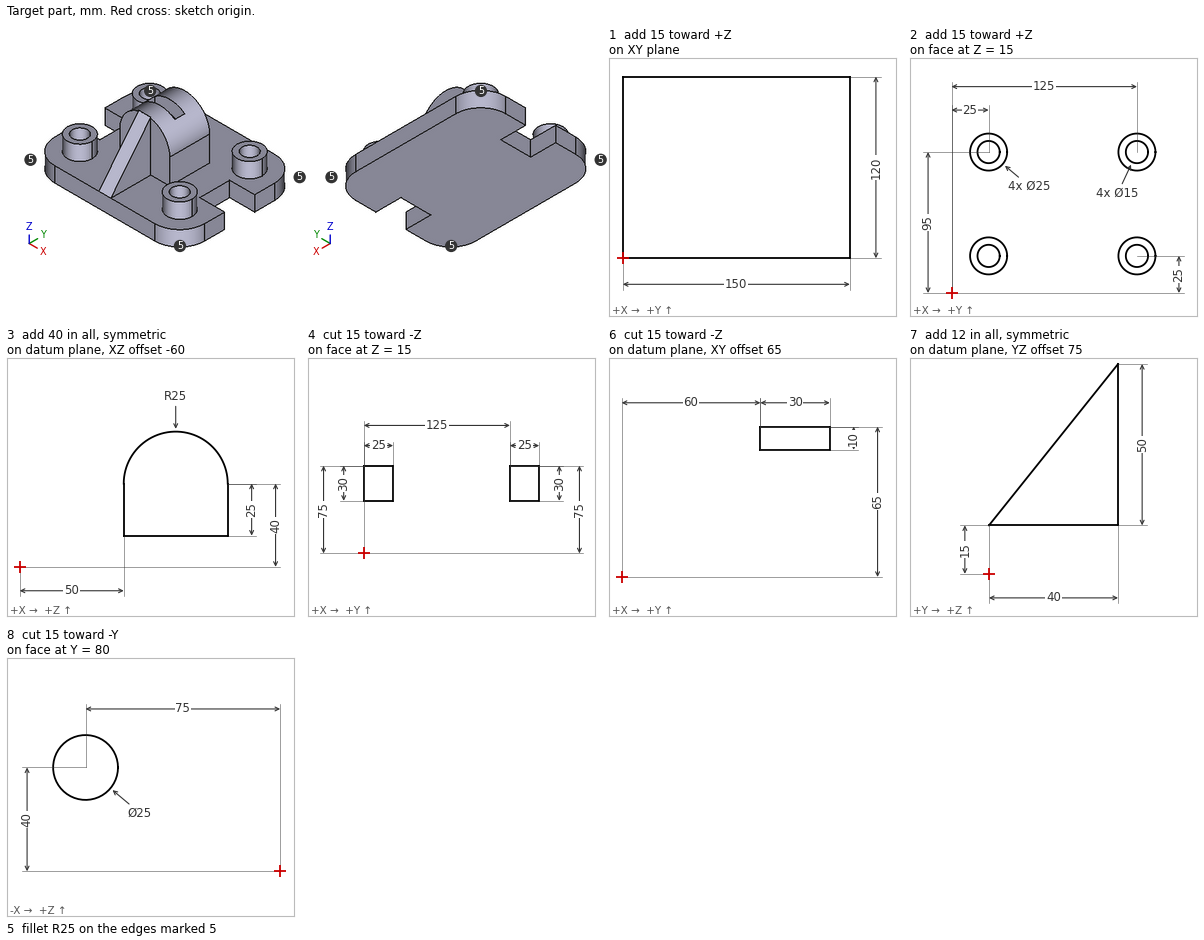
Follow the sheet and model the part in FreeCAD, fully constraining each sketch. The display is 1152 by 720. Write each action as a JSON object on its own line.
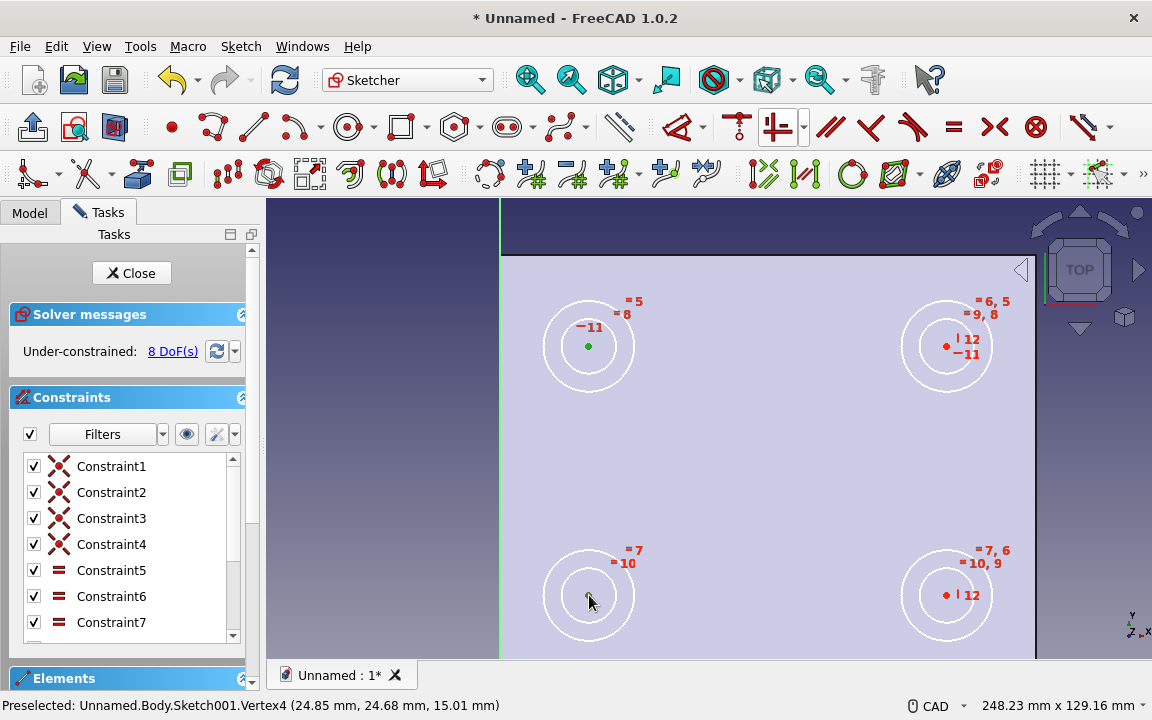
{"action": "key", "text": "v"}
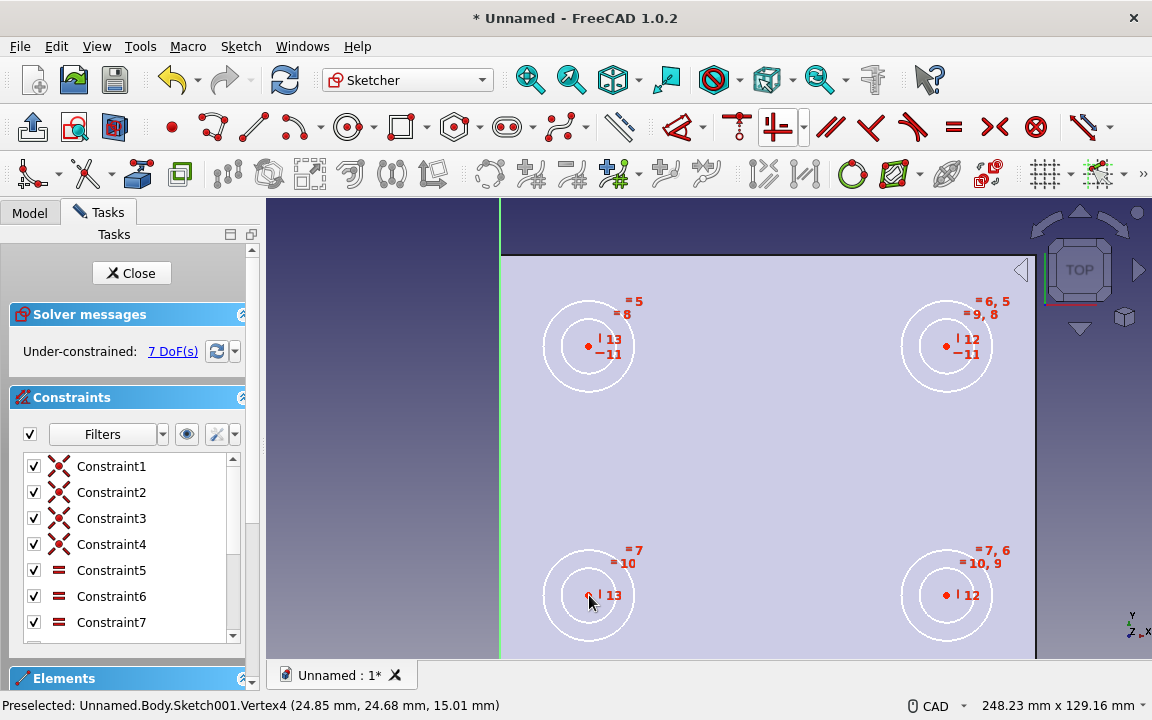
{"action": "left_click", "coordinate": [947, 595]}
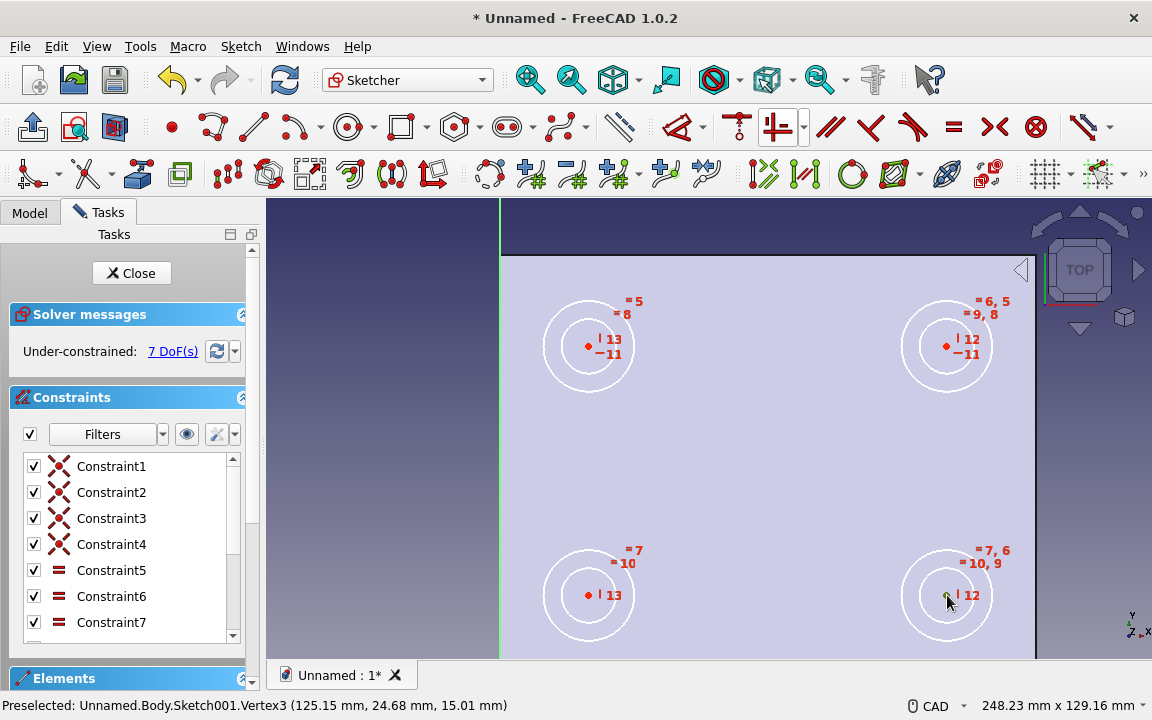
{"action": "left_click", "coordinate": [589, 595]}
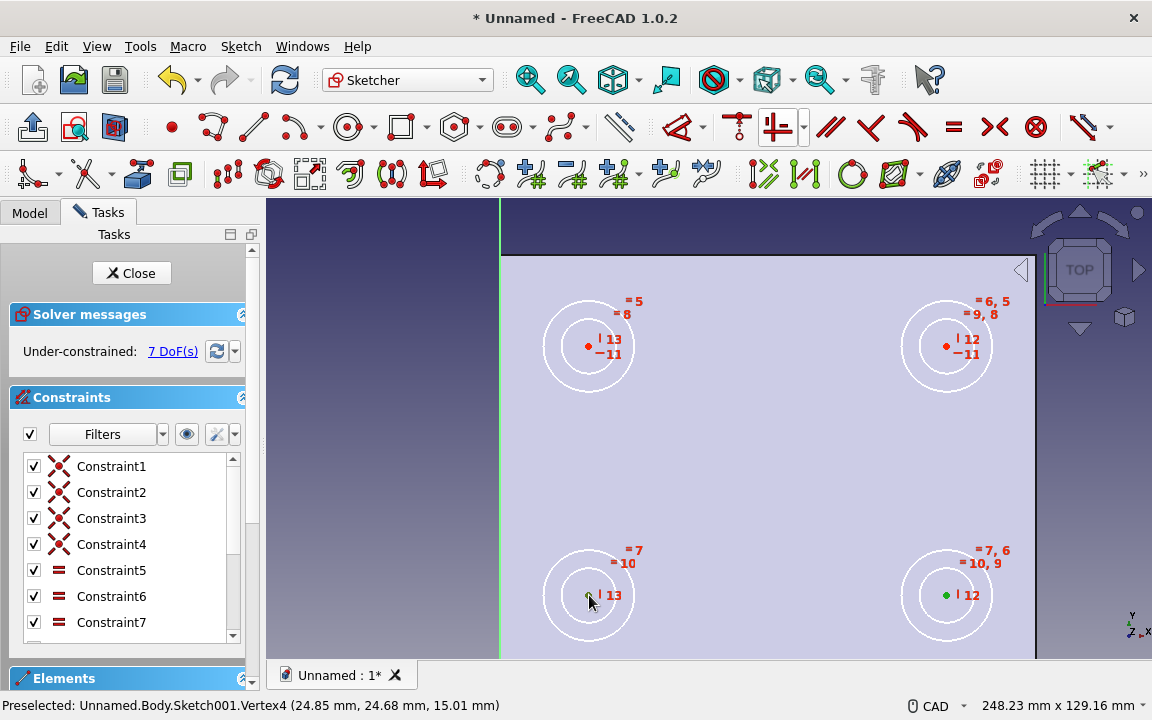
{"action": "key", "text": "h"}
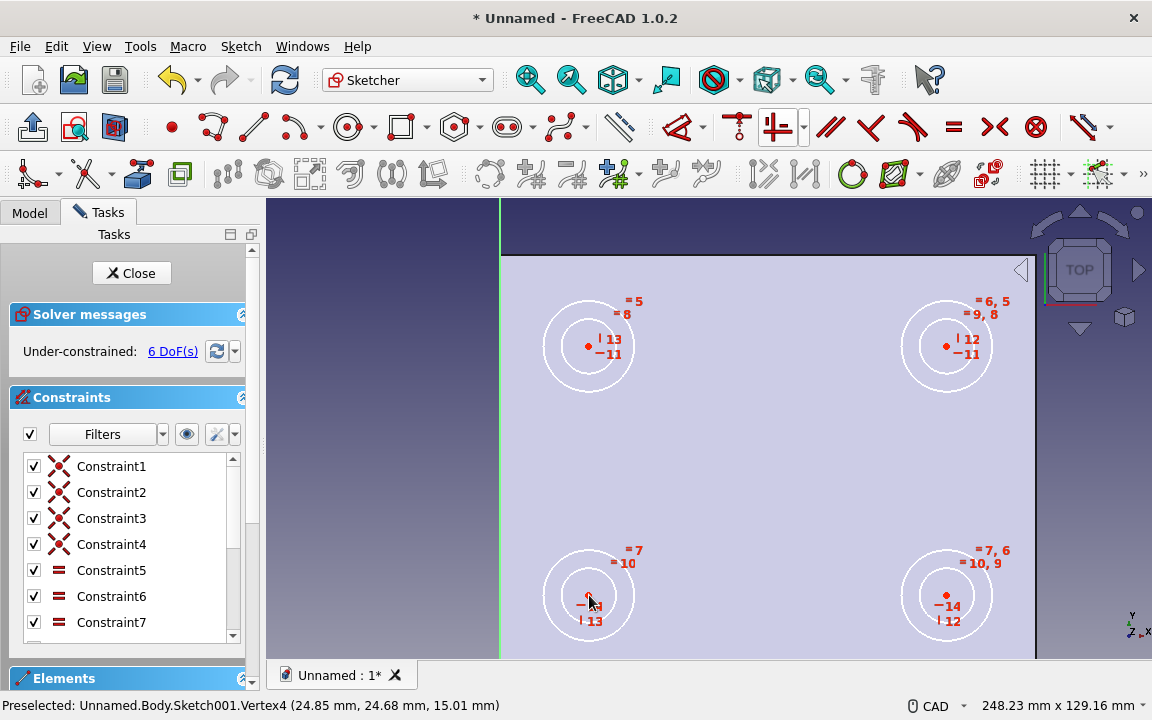
{"action": "left_click", "coordinate": [676, 128]}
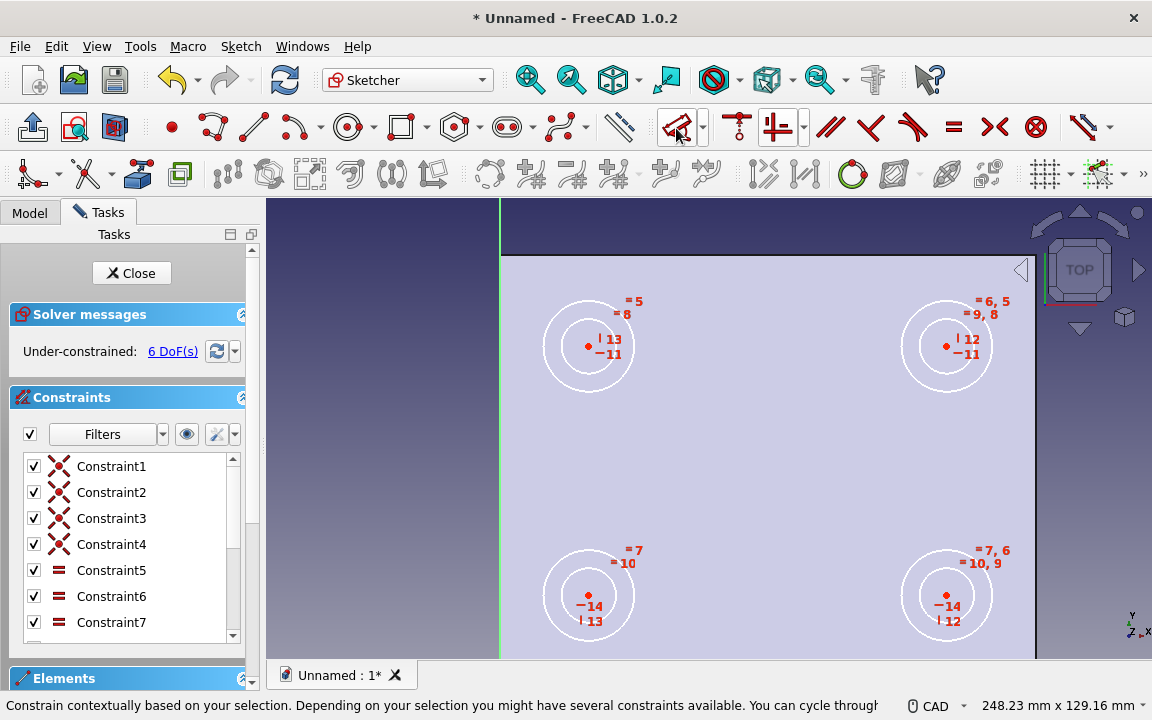
{"action": "left_click", "coordinate": [621, 314]}
{"action": "left_click", "coordinate": [644, 291]}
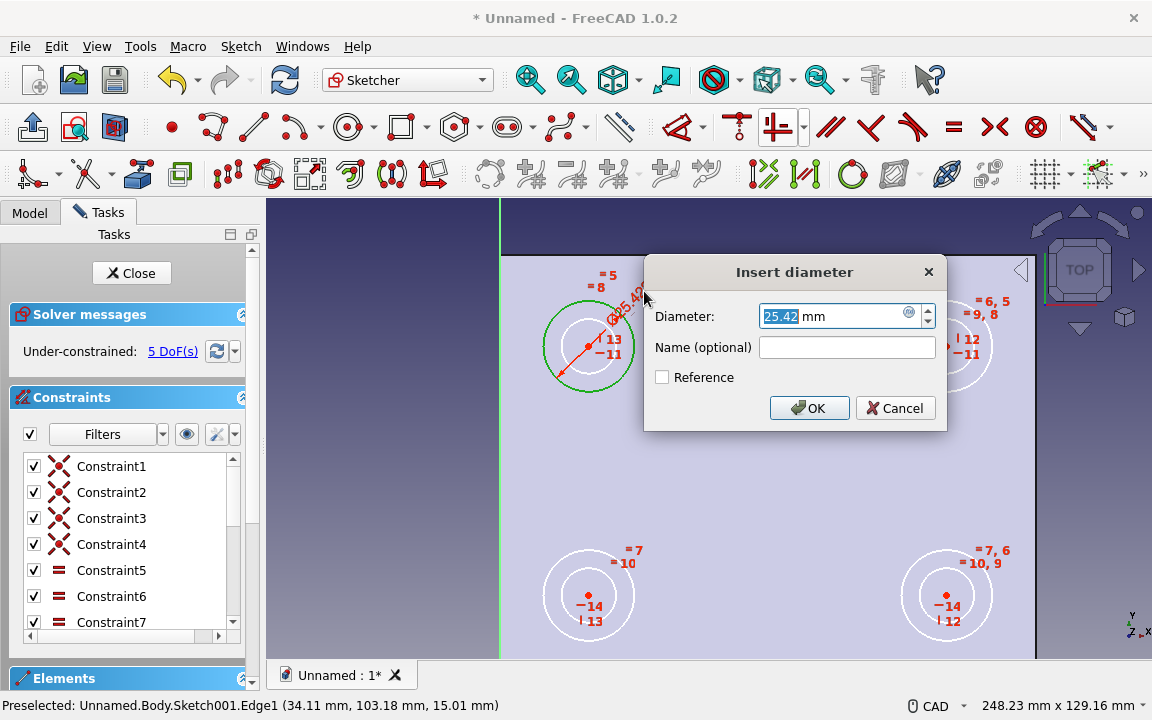
{"action": "type", "text": "25"}
{"action": "key", "text": "Return"}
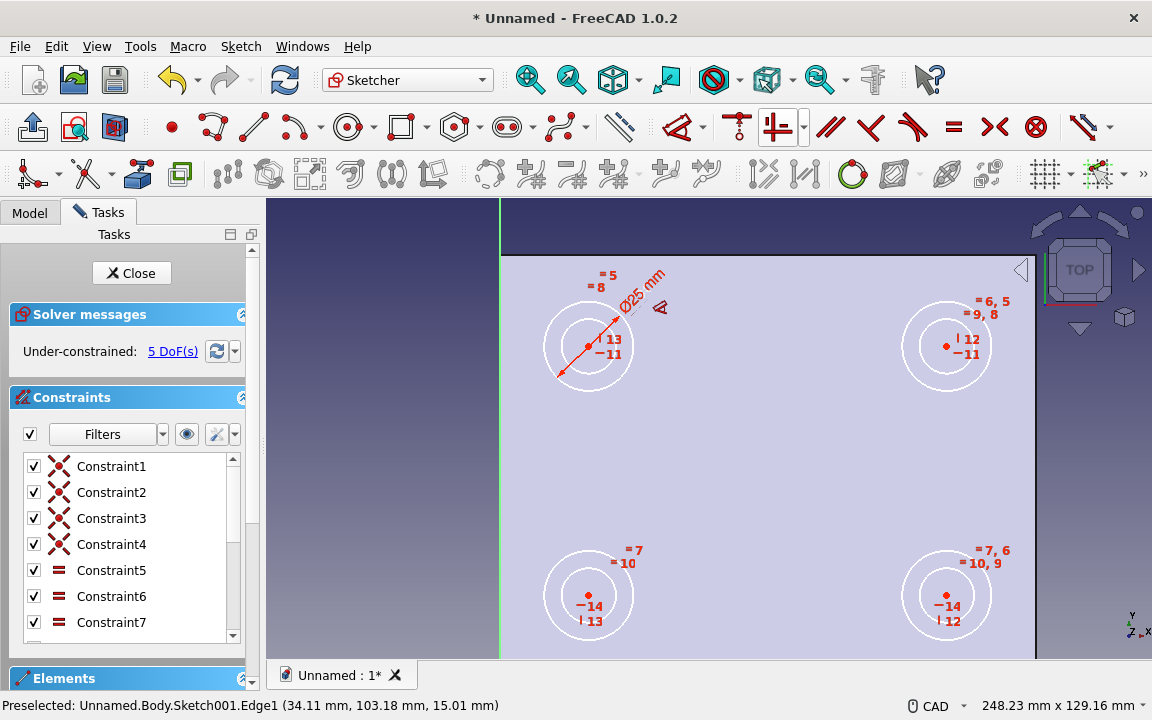
{"action": "left_click", "coordinate": [608, 327]}
{"action": "left_click", "coordinate": [646, 329]}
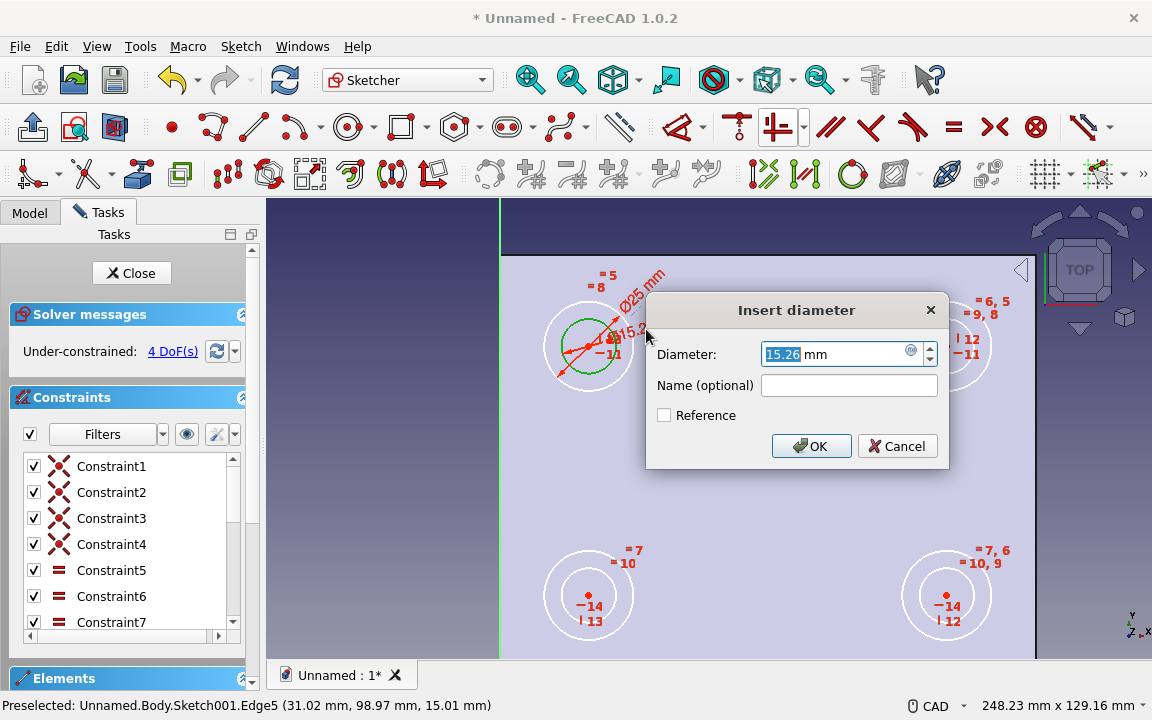
{"action": "type", "text": "15"}
{"action": "key", "text": "Return"}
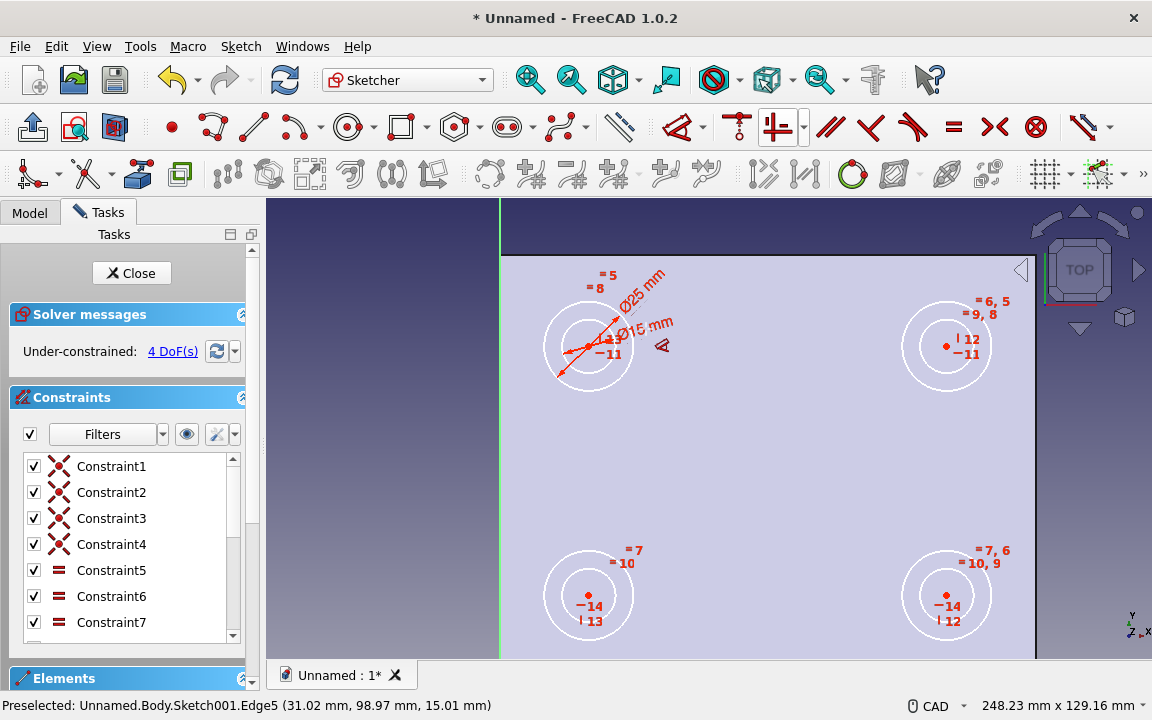
{"action": "left_click", "coordinate": [589, 346]}
{"action": "left_click", "coordinate": [524, 312]}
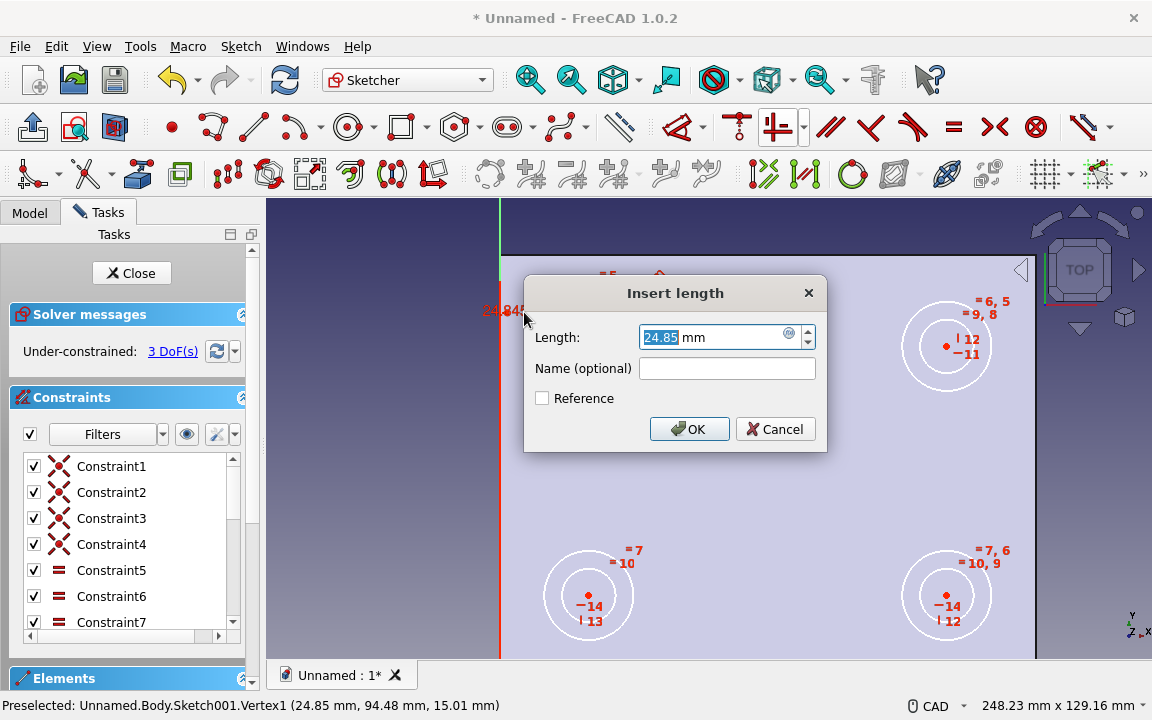
{"action": "type", "text": "25"}
{"action": "key", "text": "Return"}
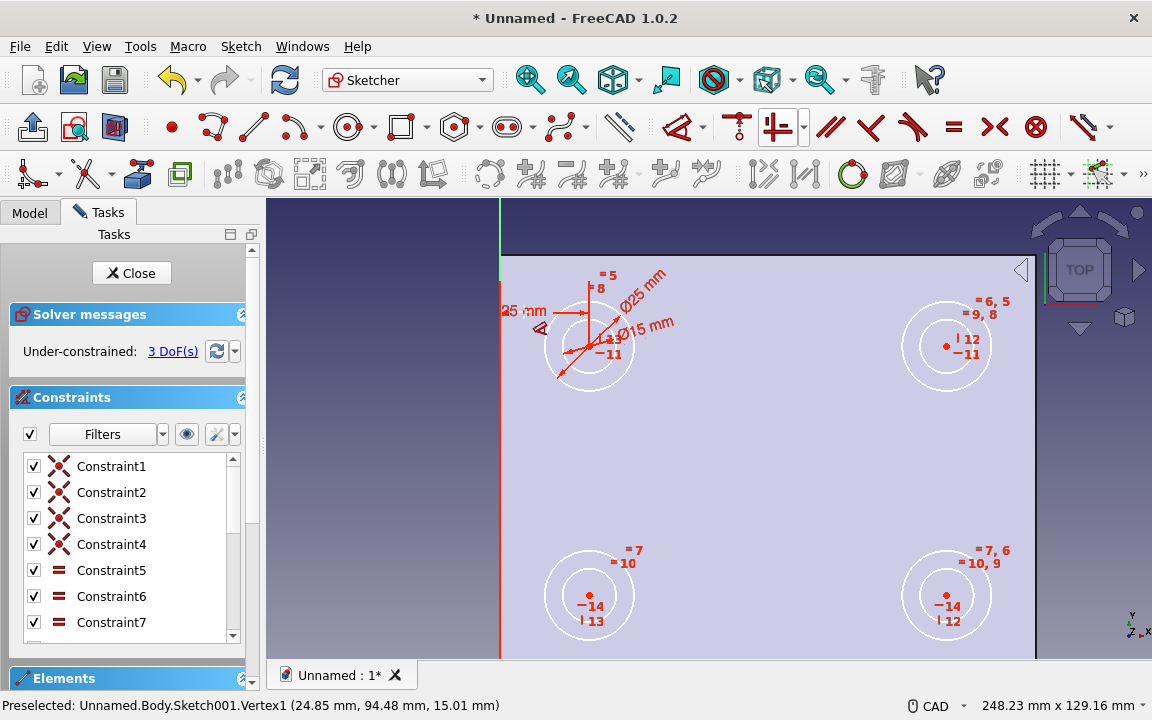
{"action": "left_click", "coordinate": [589, 346]}
{"action": "left_click", "coordinate": [466, 489]}